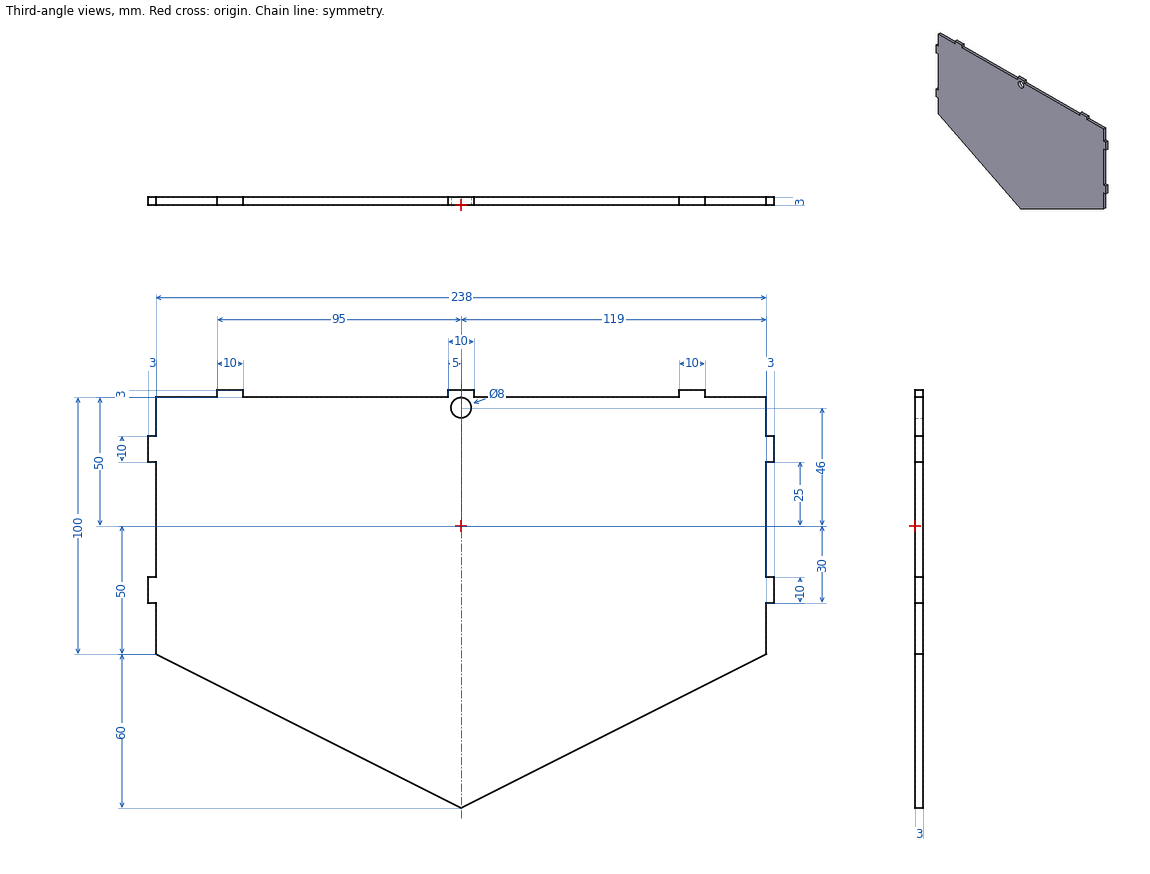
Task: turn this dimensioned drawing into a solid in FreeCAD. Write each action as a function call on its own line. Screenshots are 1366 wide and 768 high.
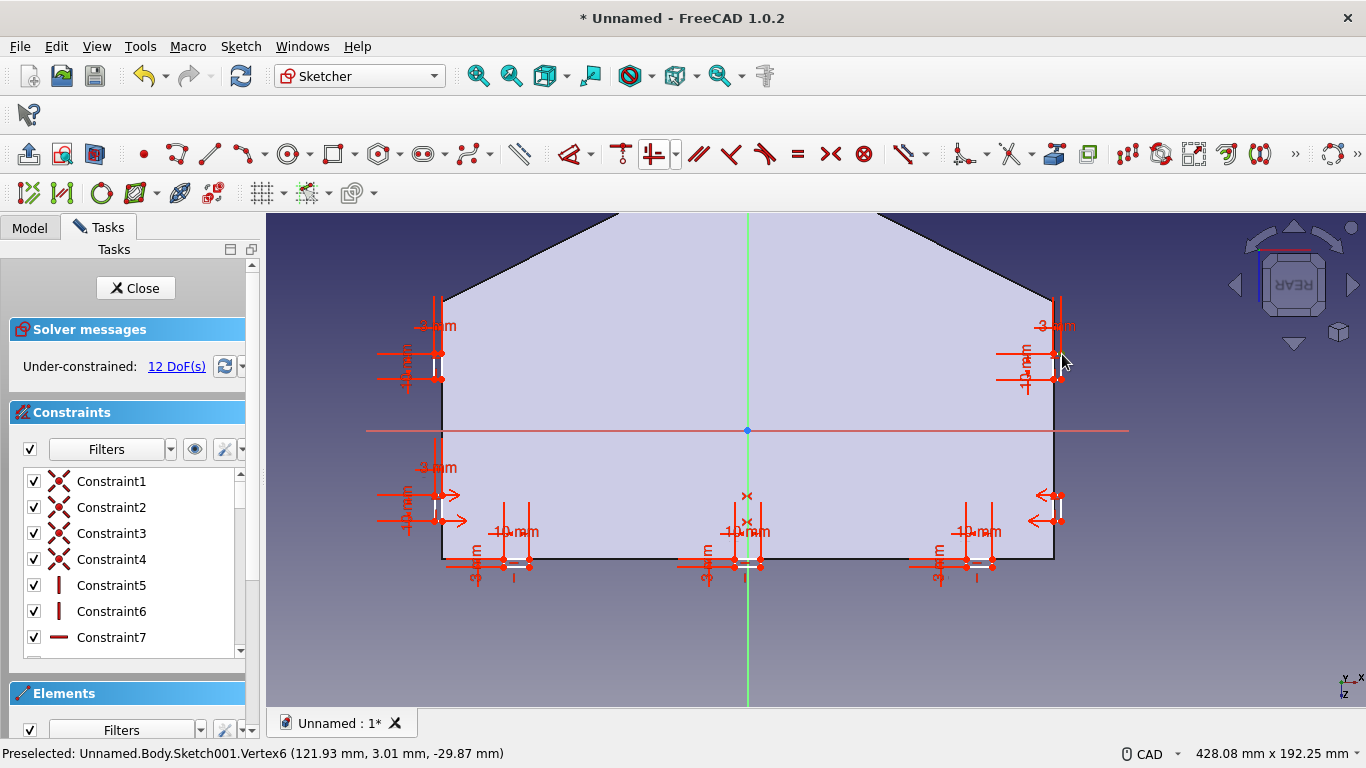
scroll(434, 354, up, 3)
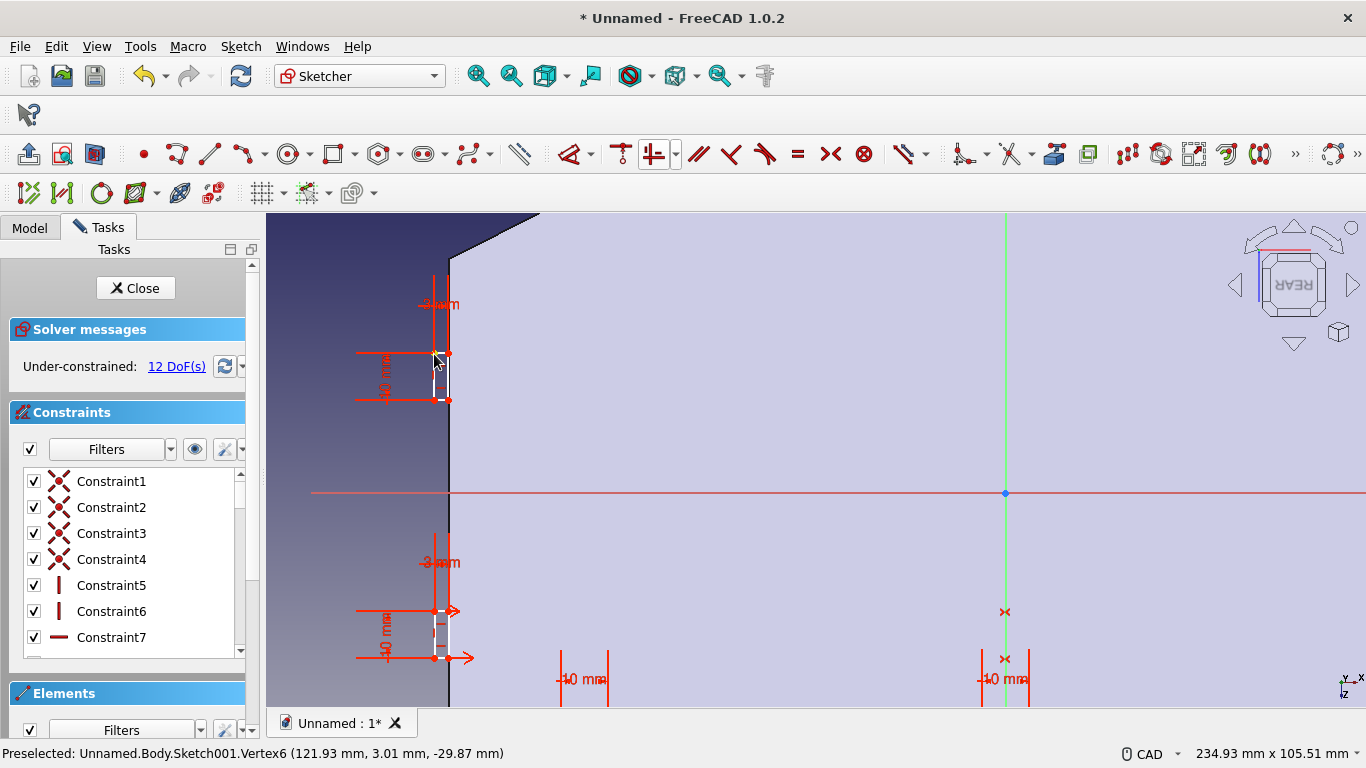
click(434, 353)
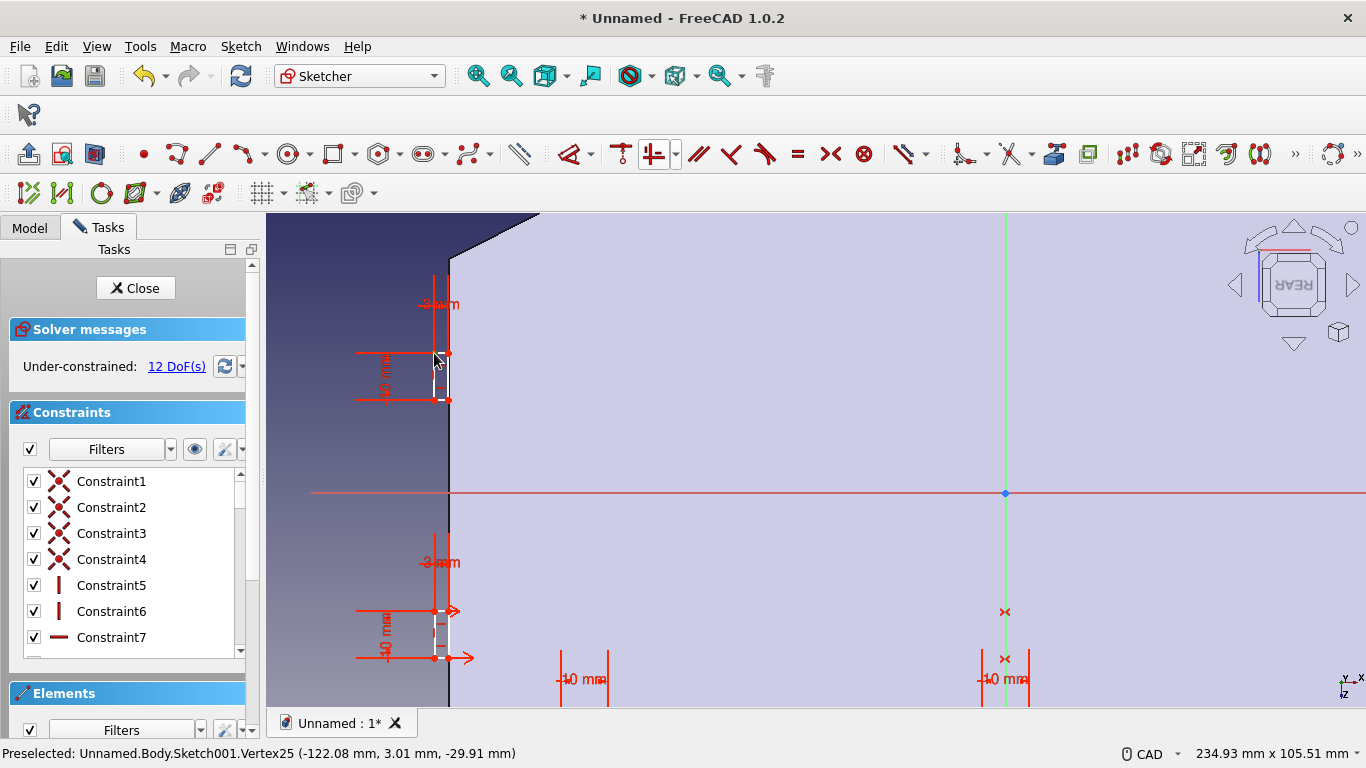
click(1006, 648)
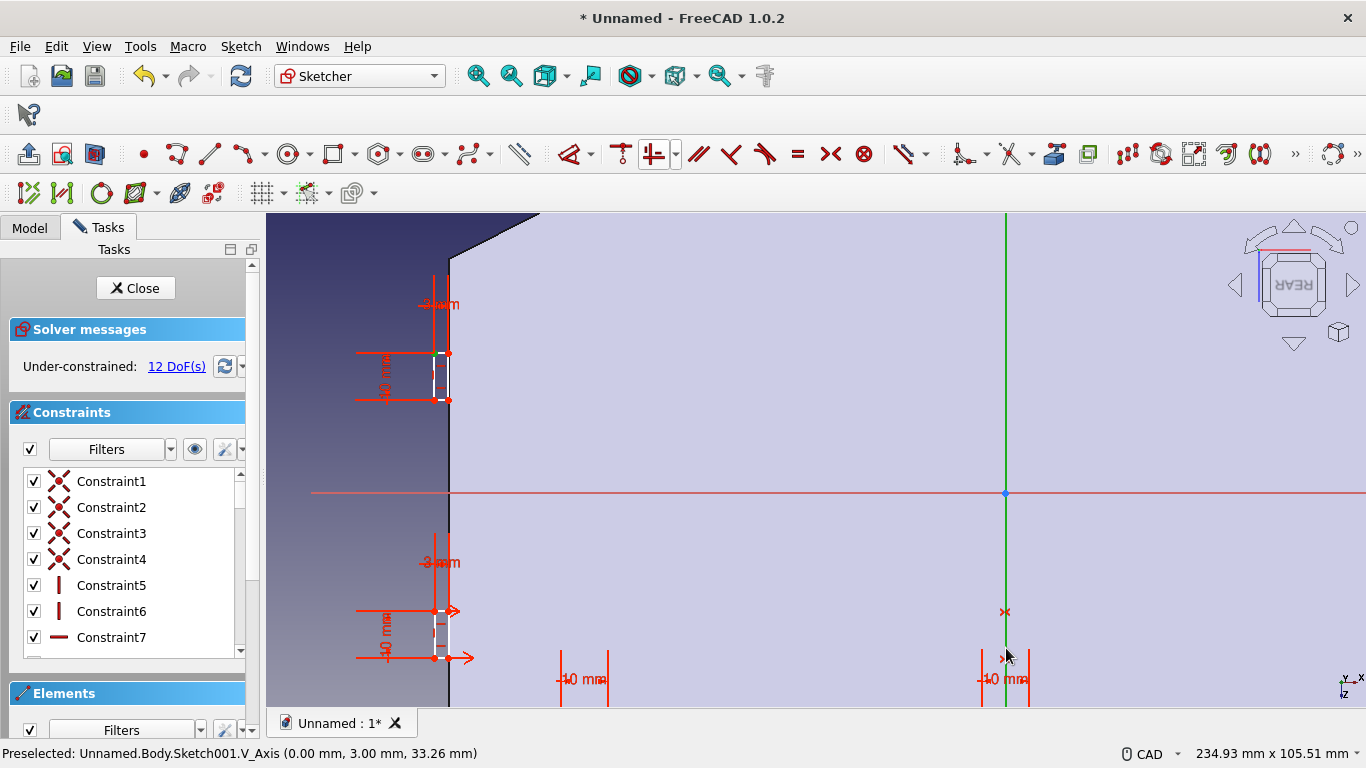
click(831, 154)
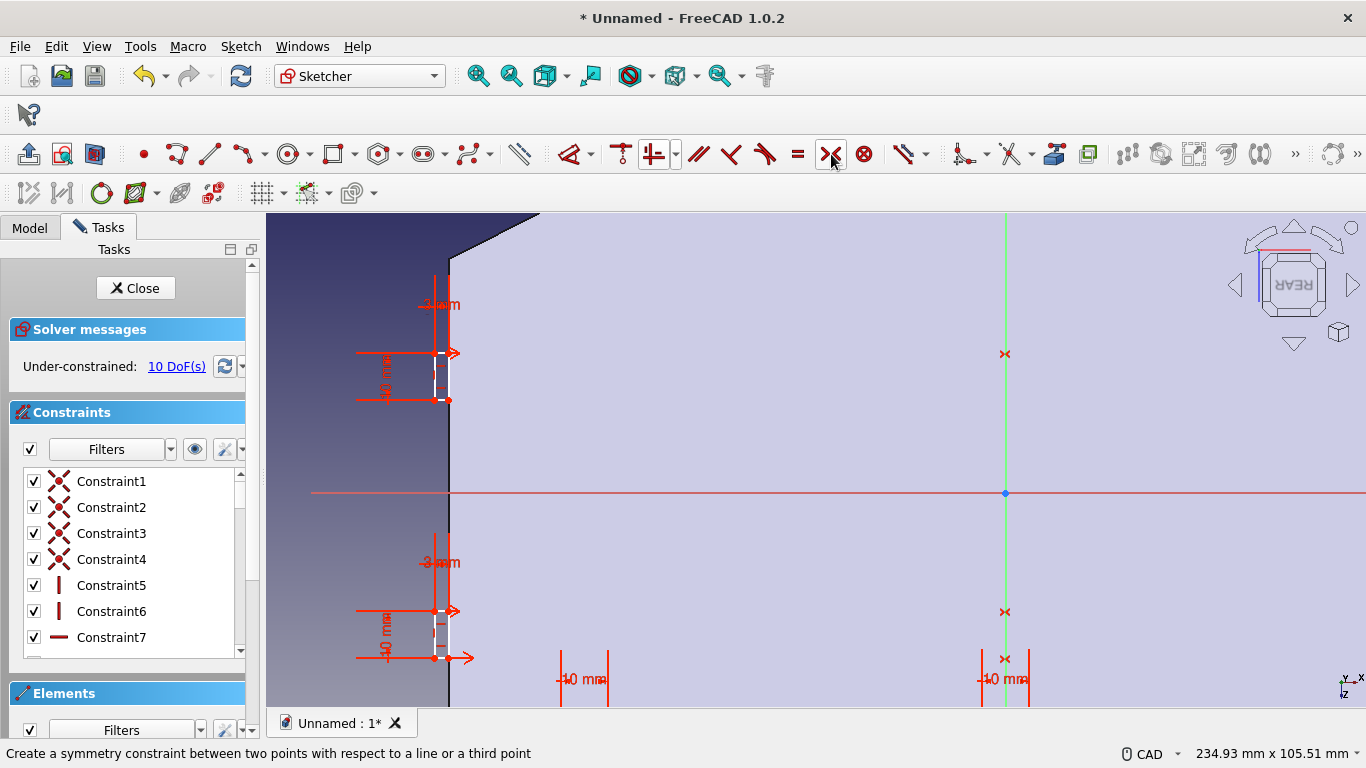
scroll(433, 354, down, 3)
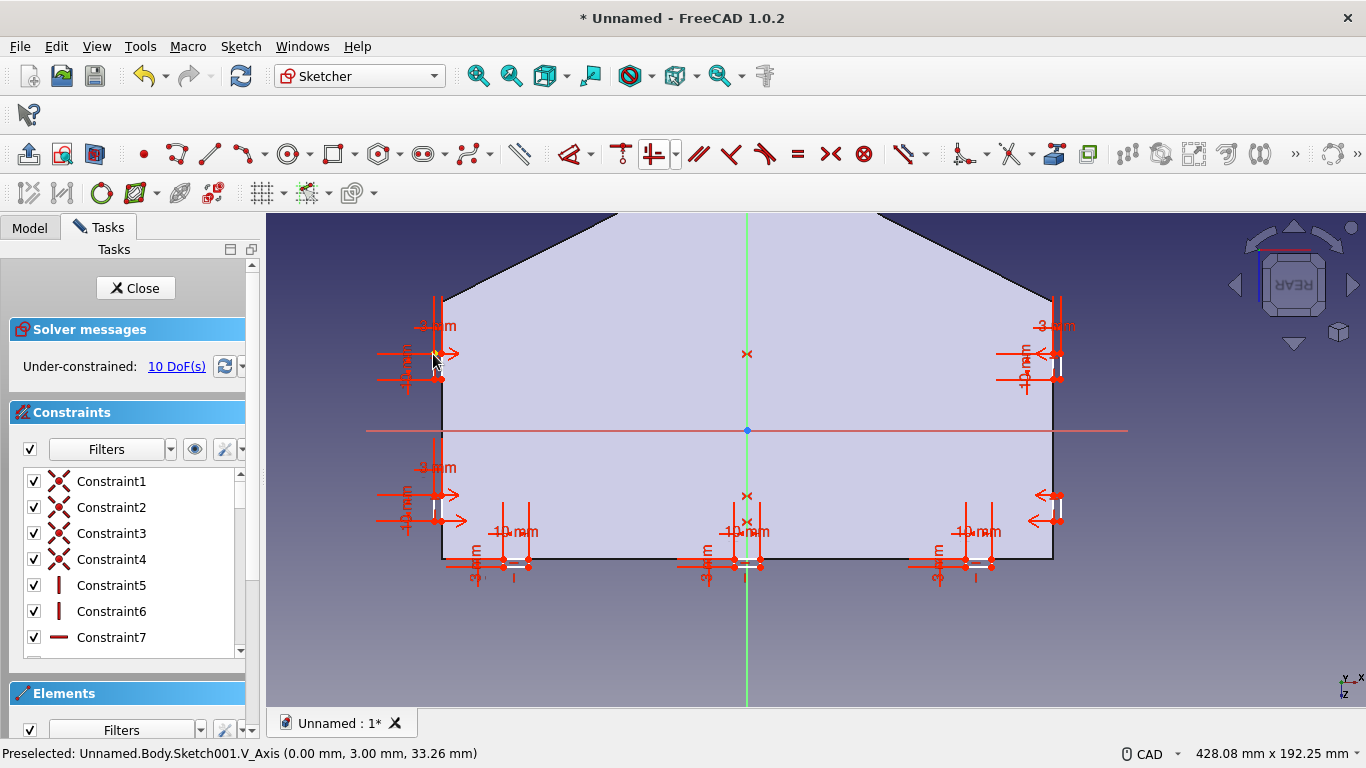
scroll(529, 559, up, 3)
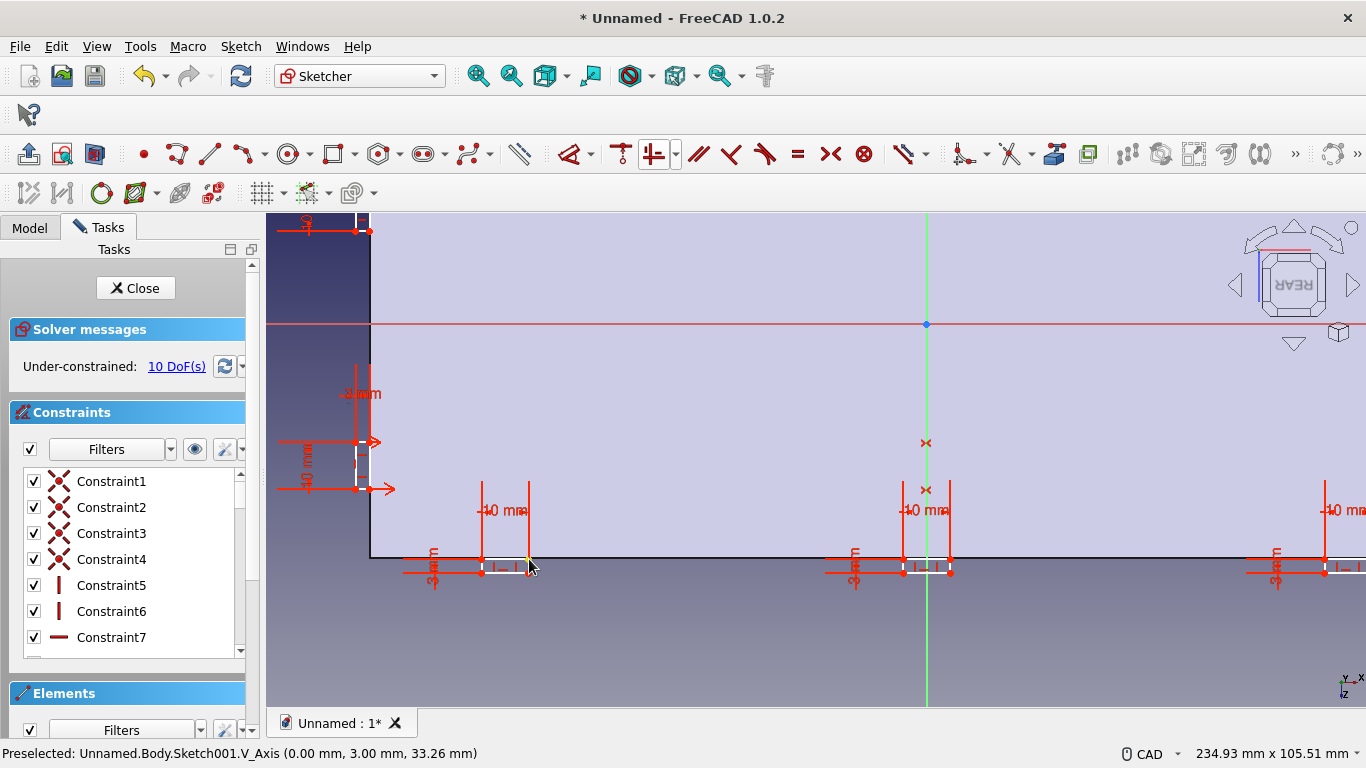
click(529, 559)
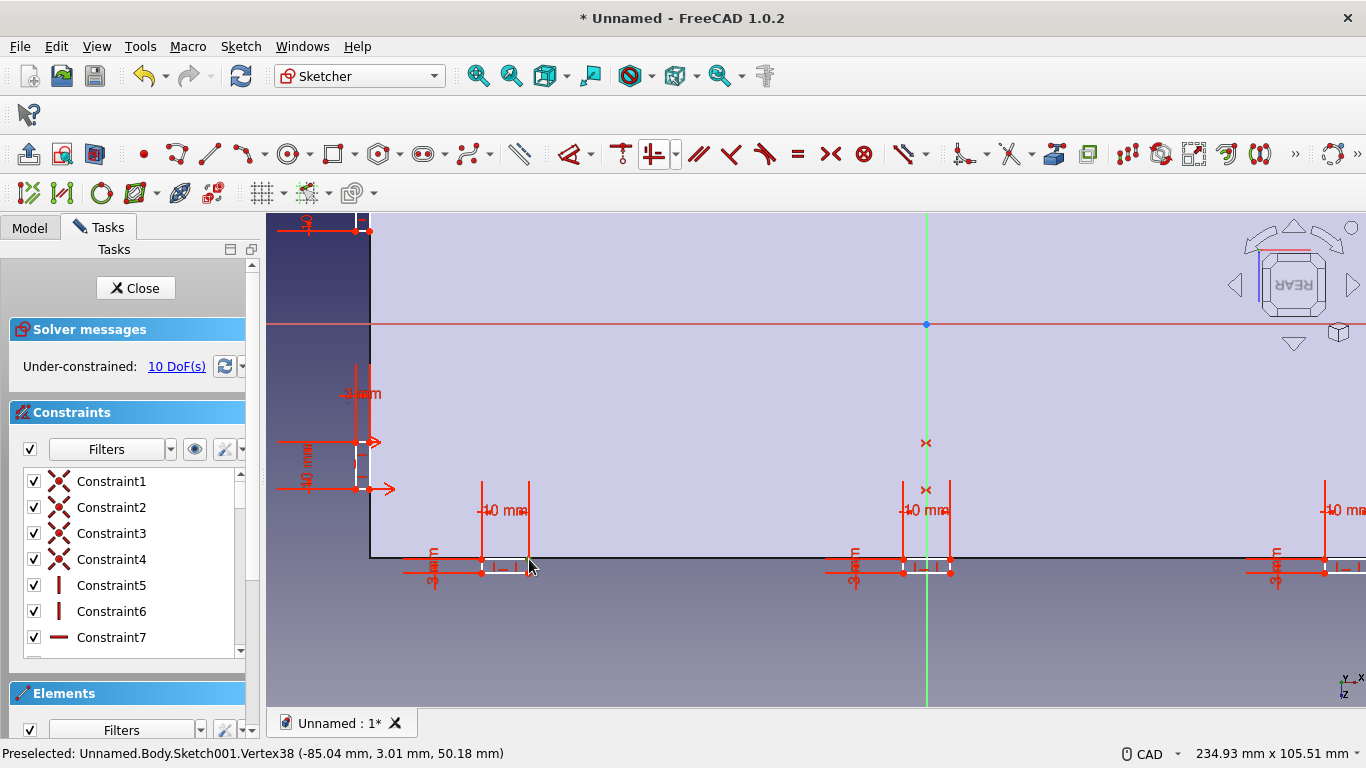
scroll(529, 559, down, 3)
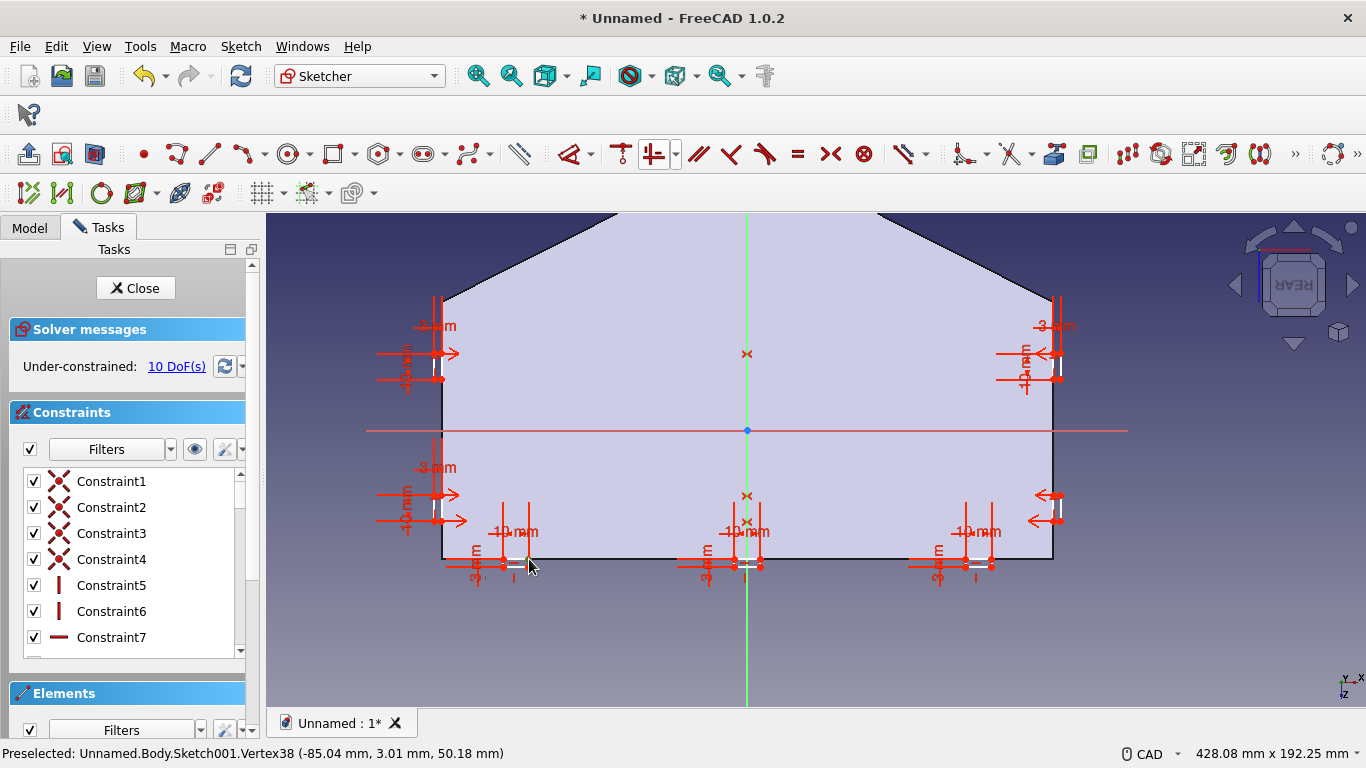
scroll(966, 559, up, 3)